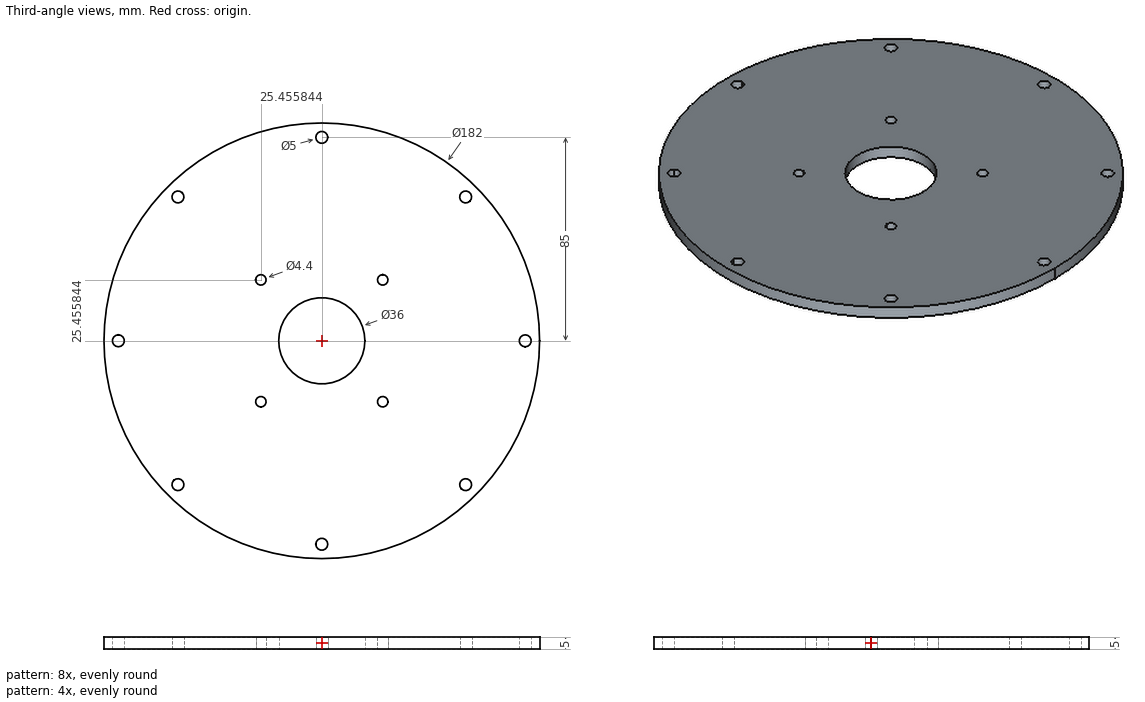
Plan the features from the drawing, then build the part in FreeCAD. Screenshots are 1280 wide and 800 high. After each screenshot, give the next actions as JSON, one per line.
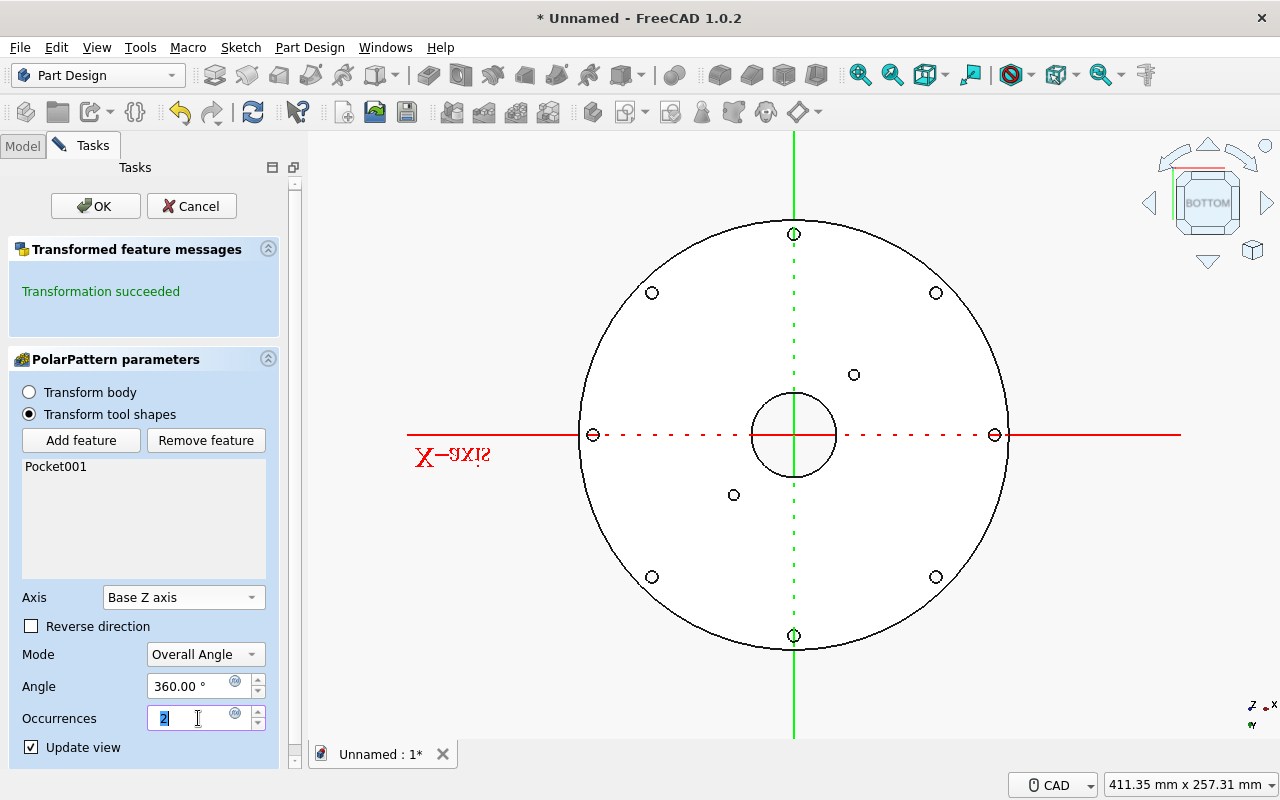
{"action": "type", "text": "4"}
{"action": "key", "text": "Tab"}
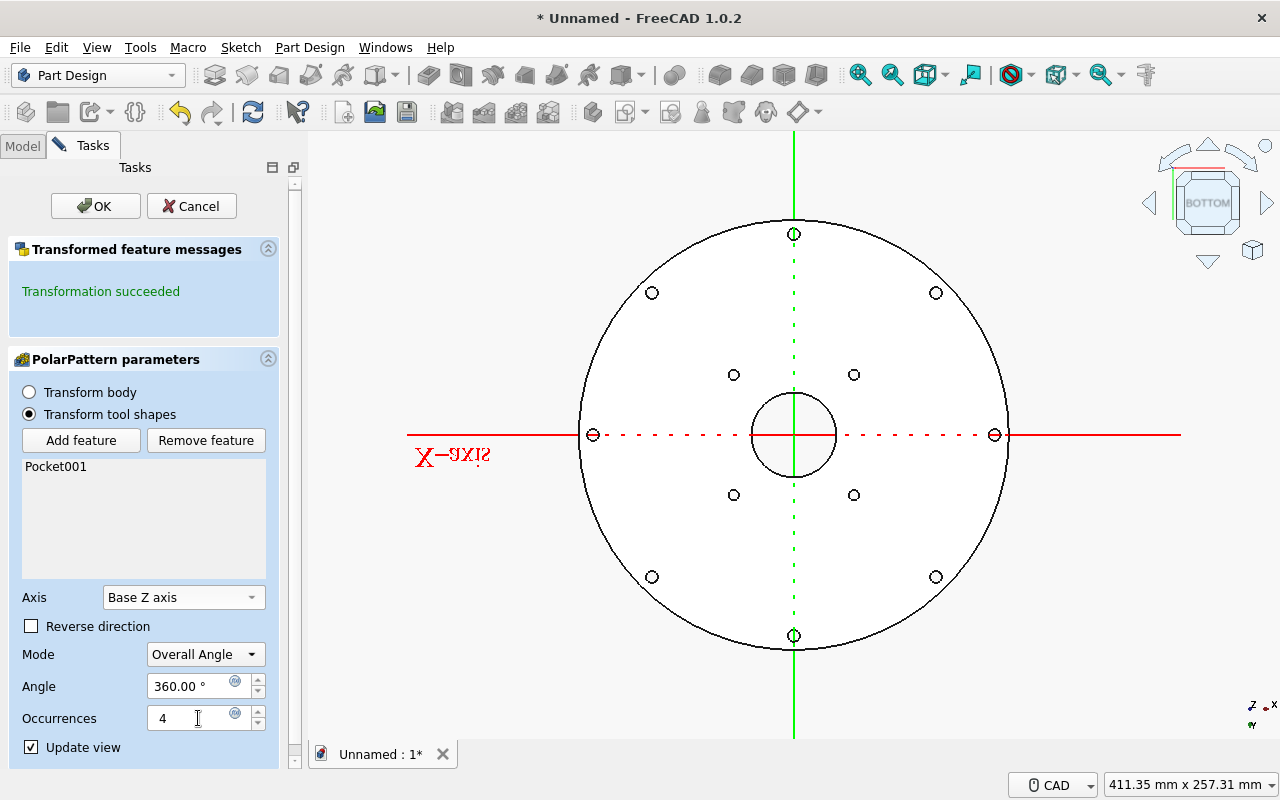
{"action": "left_click", "coordinate": [96, 206]}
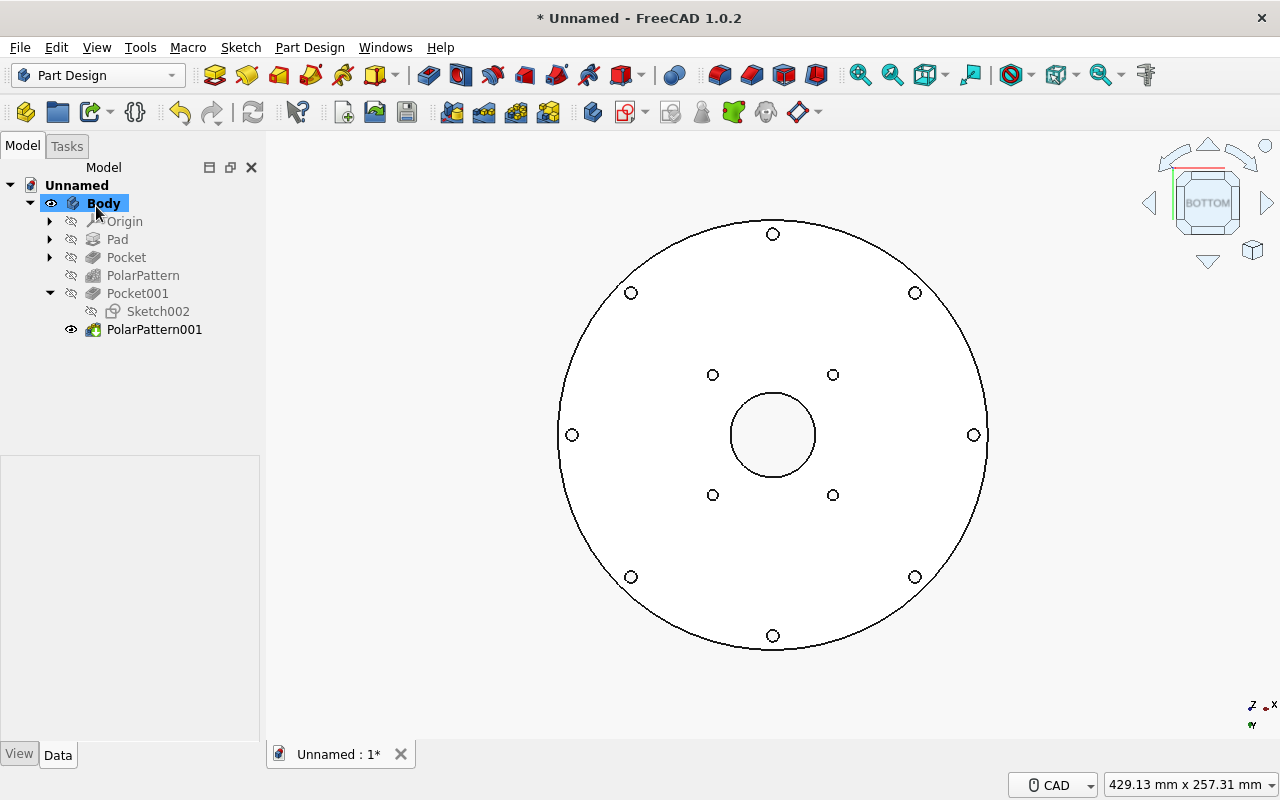
{"action": "key", "text": "0"}